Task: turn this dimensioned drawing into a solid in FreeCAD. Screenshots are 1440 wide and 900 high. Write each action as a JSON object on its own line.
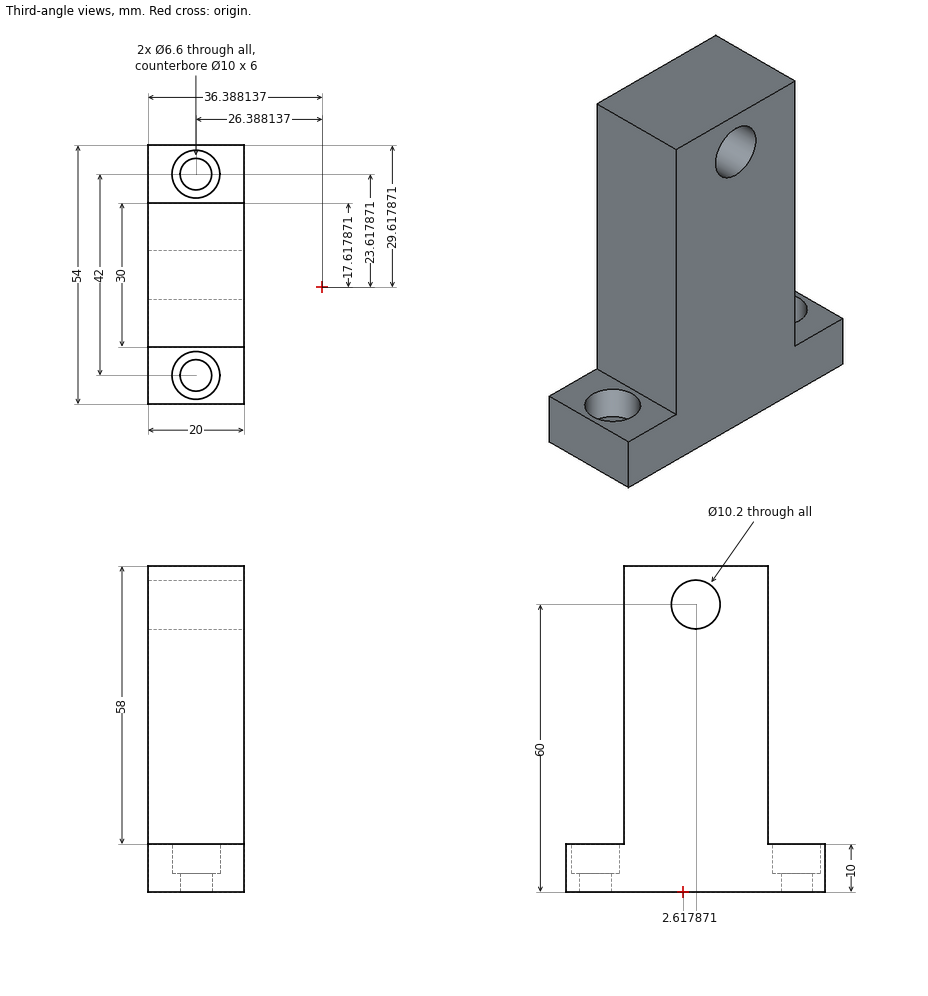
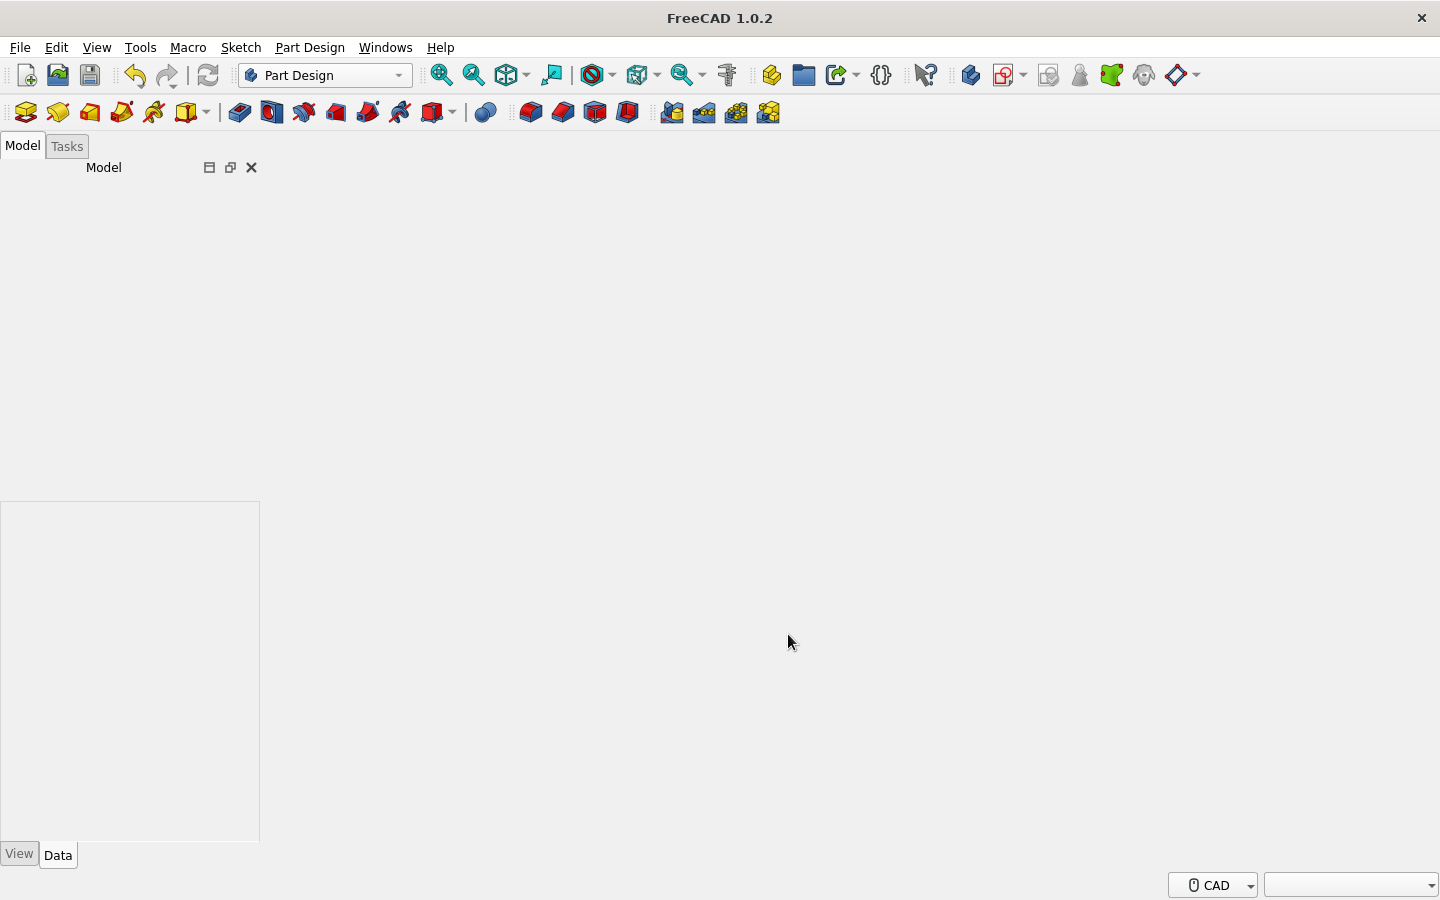
{"action": "left_click", "coordinate": [26, 76]}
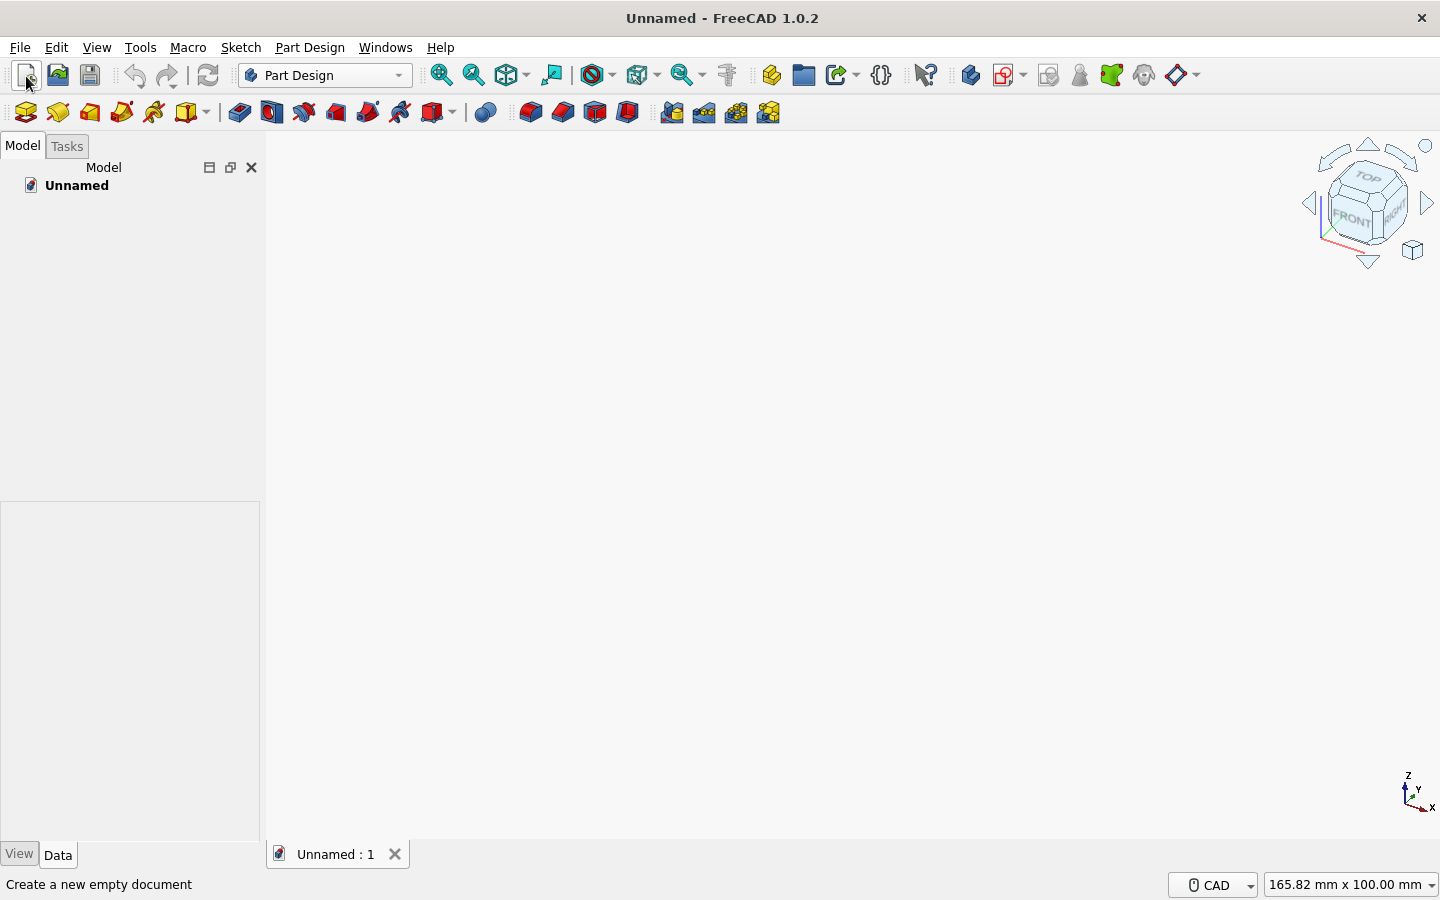
{"action": "left_click", "coordinate": [1004, 76]}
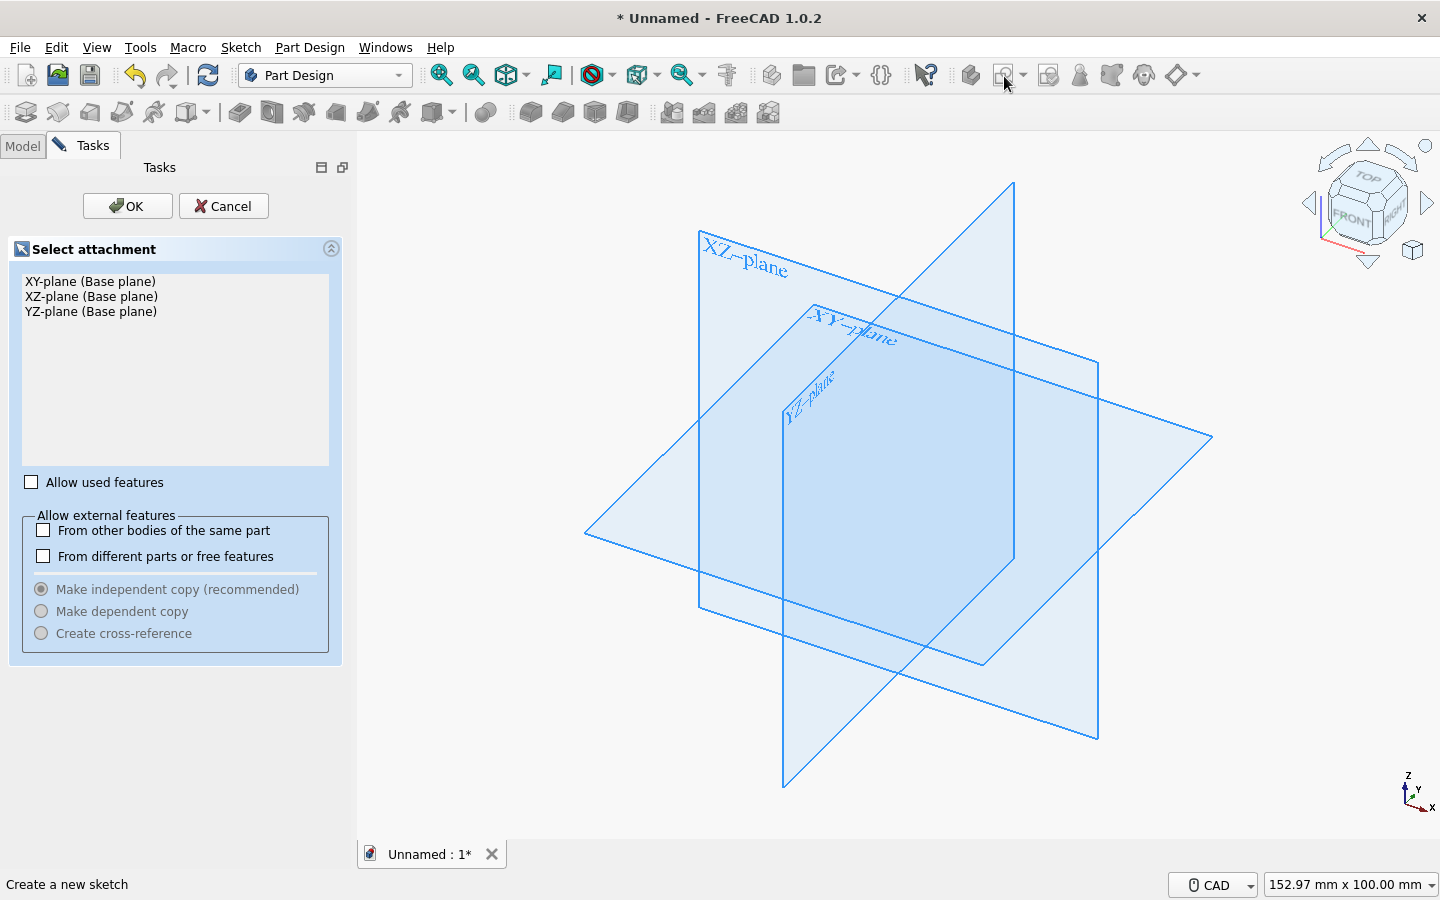
{"action": "left_click", "coordinate": [82, 282]}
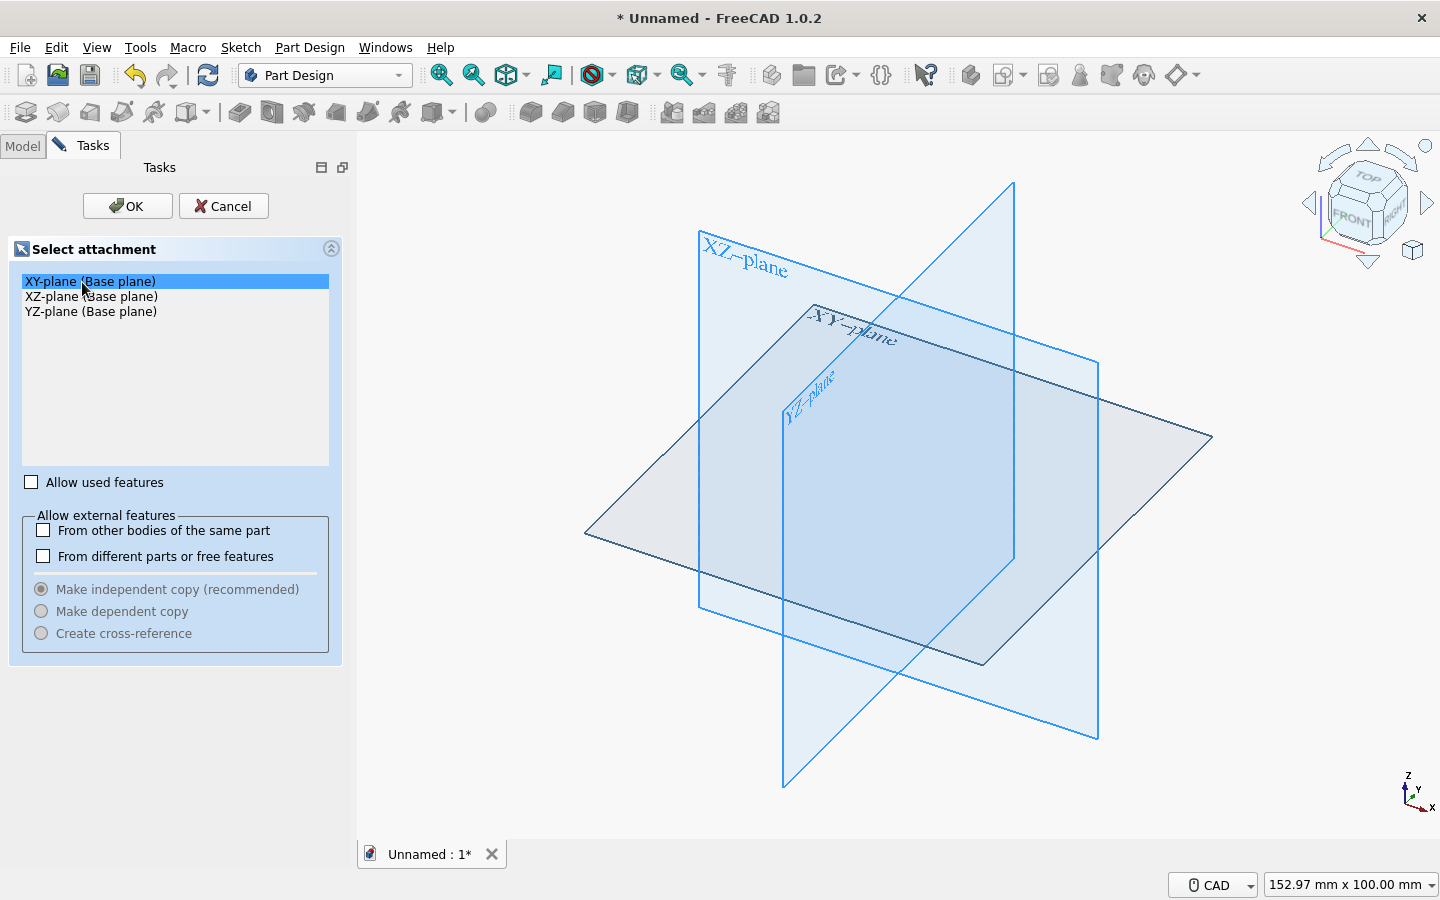
{"action": "left_click", "coordinate": [128, 206]}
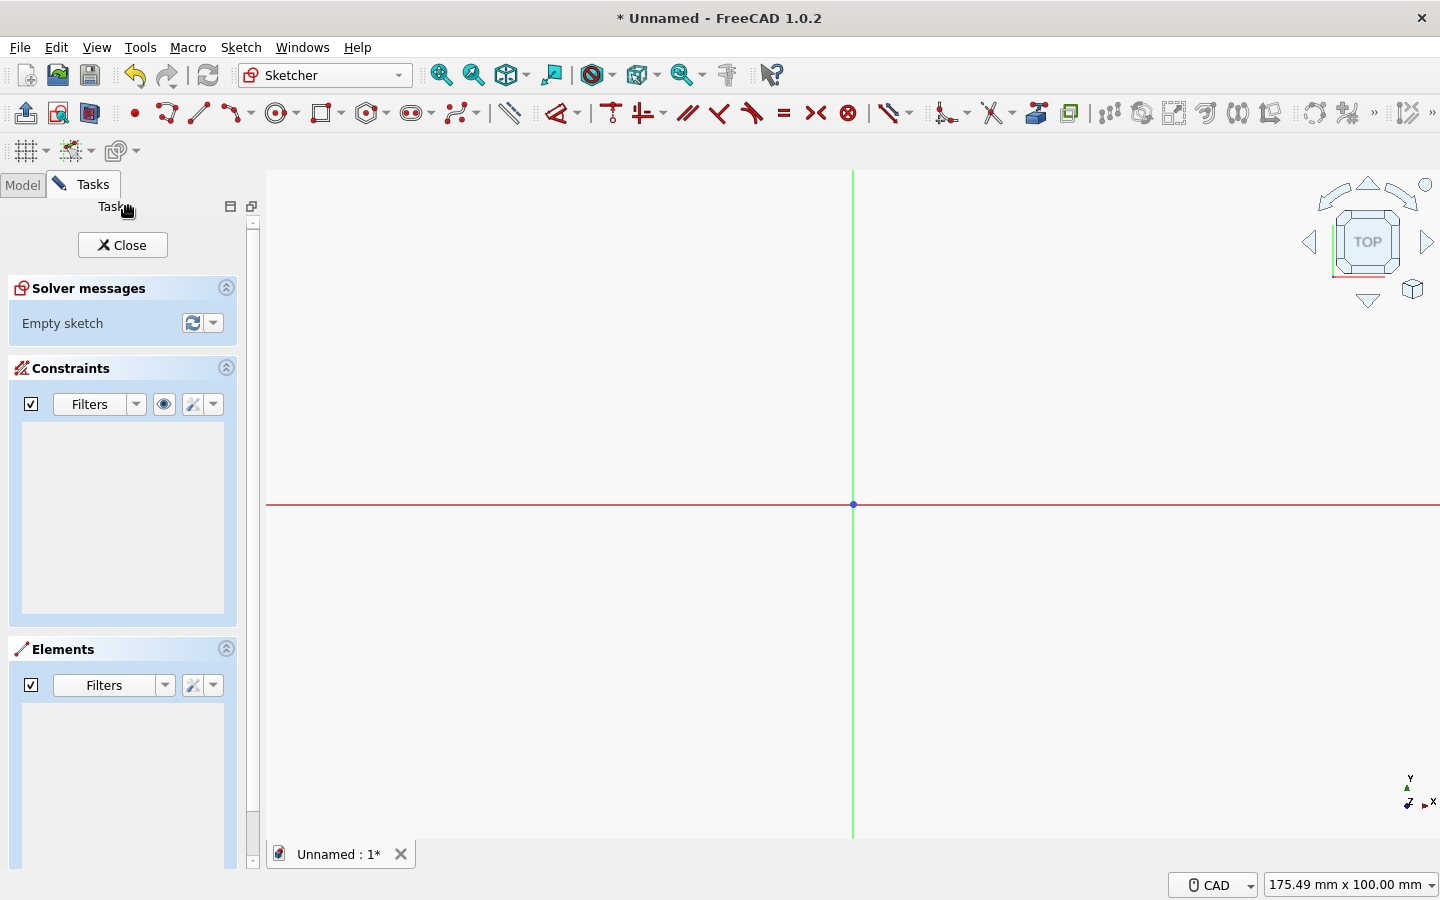
{"action": "left_click", "coordinate": [322, 114]}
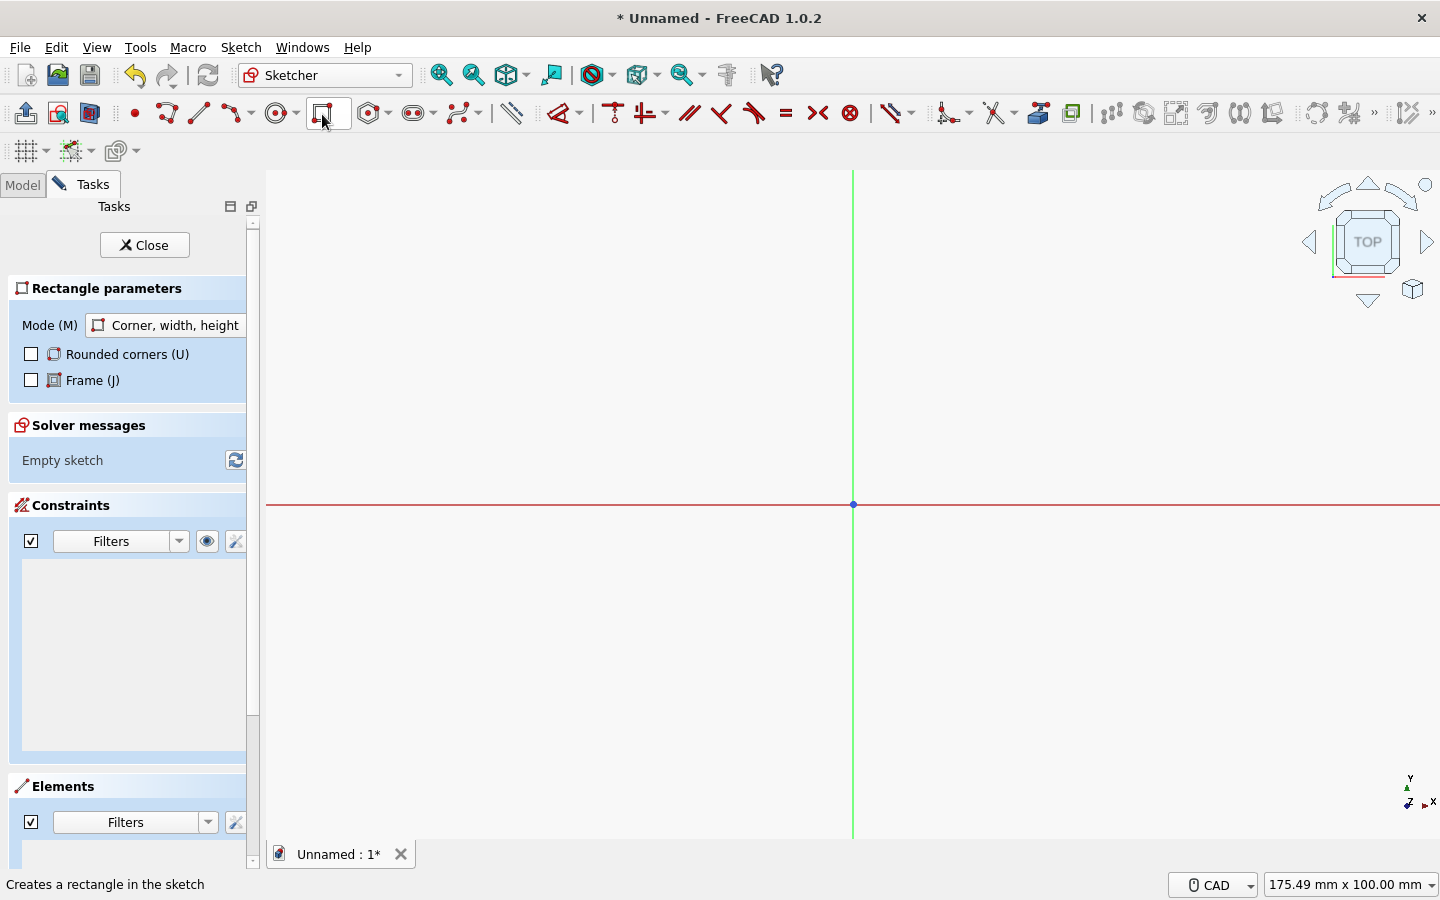
{"action": "left_click", "coordinate": [610, 306]}
{"action": "left_click", "coordinate": [743, 668]}
{"action": "key", "text": "Escape"}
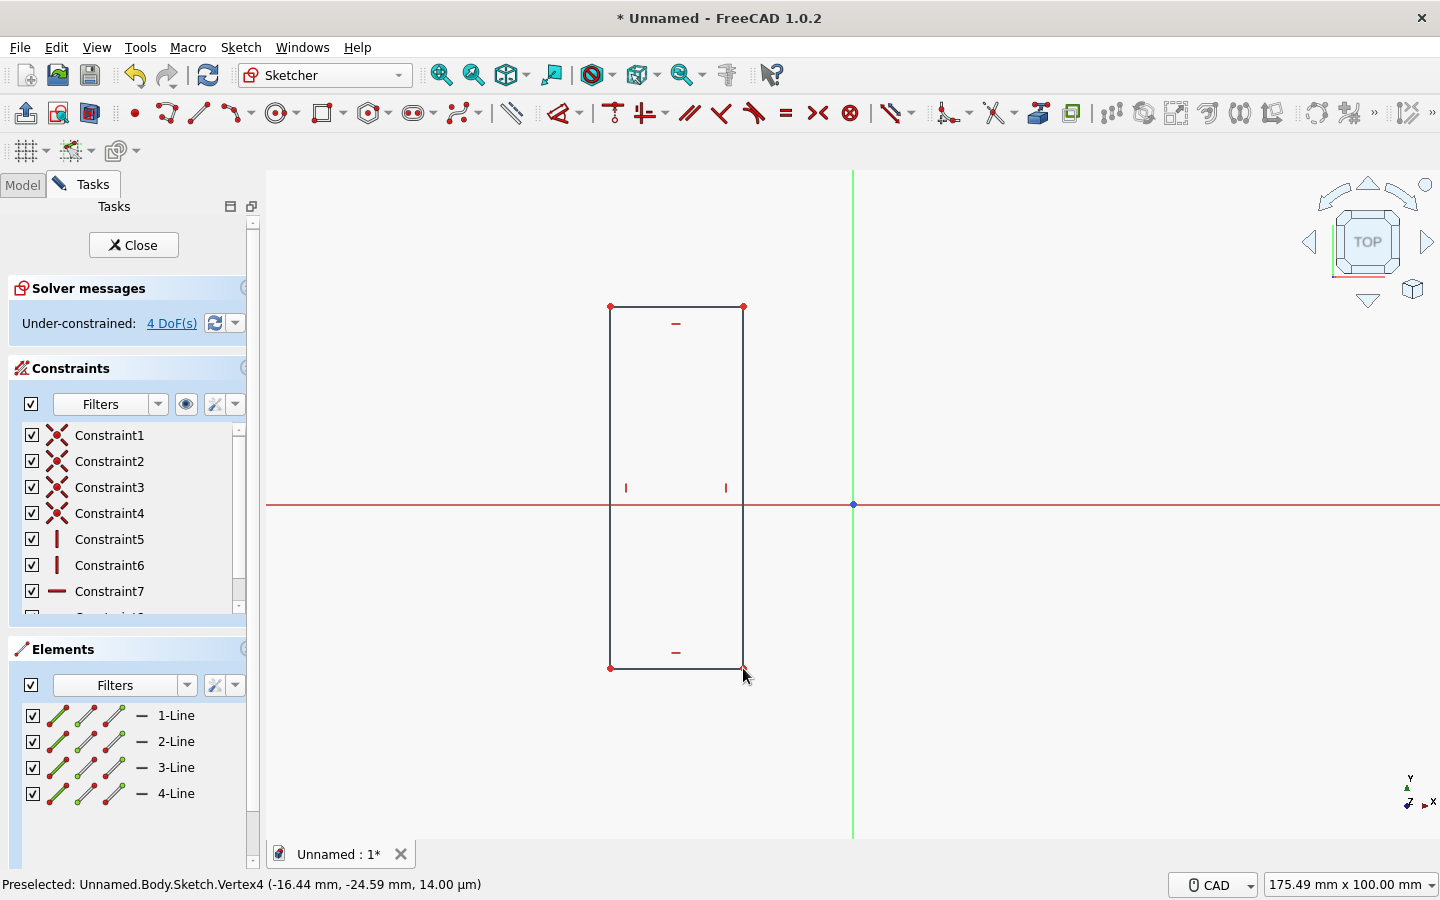
{"action": "left_click", "coordinate": [610, 416]}